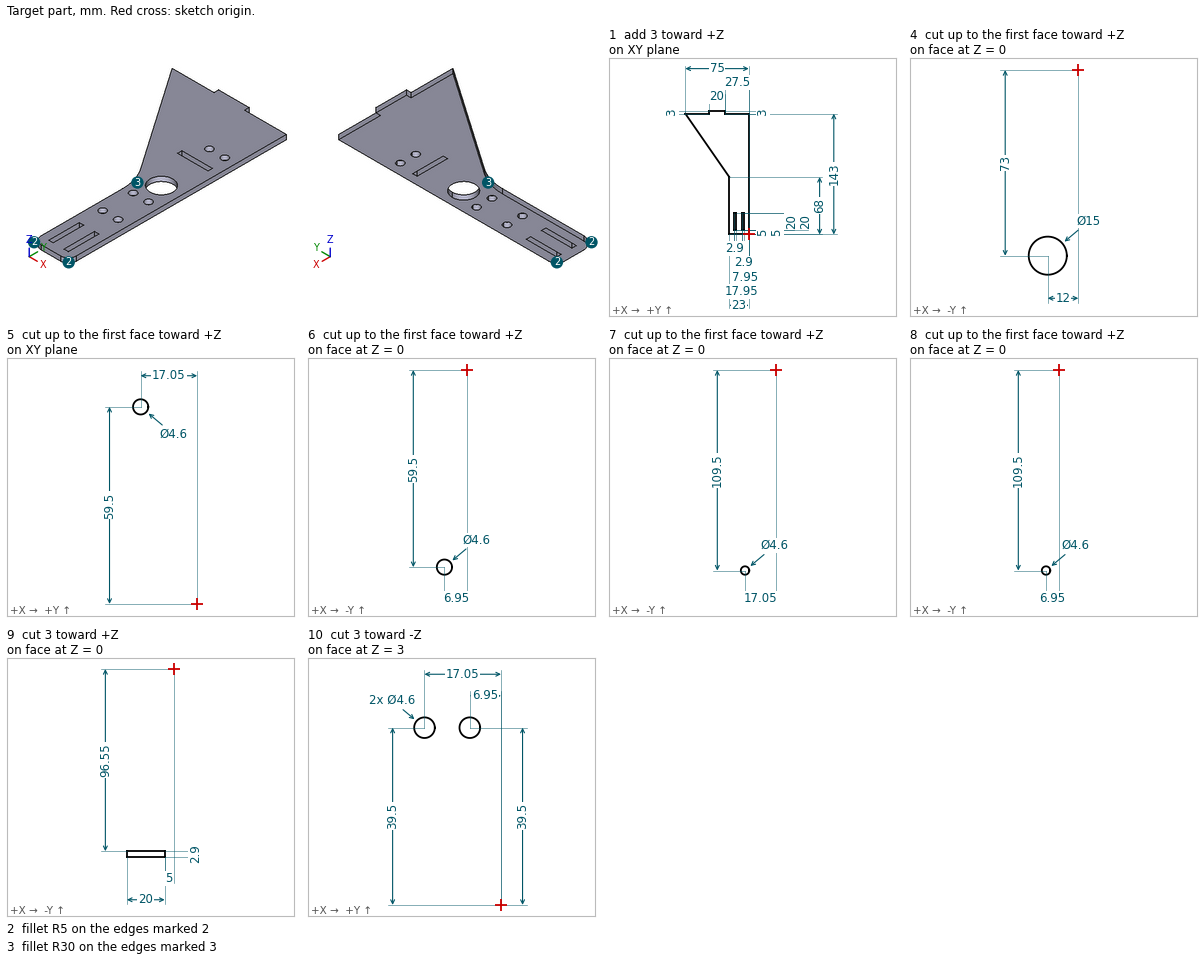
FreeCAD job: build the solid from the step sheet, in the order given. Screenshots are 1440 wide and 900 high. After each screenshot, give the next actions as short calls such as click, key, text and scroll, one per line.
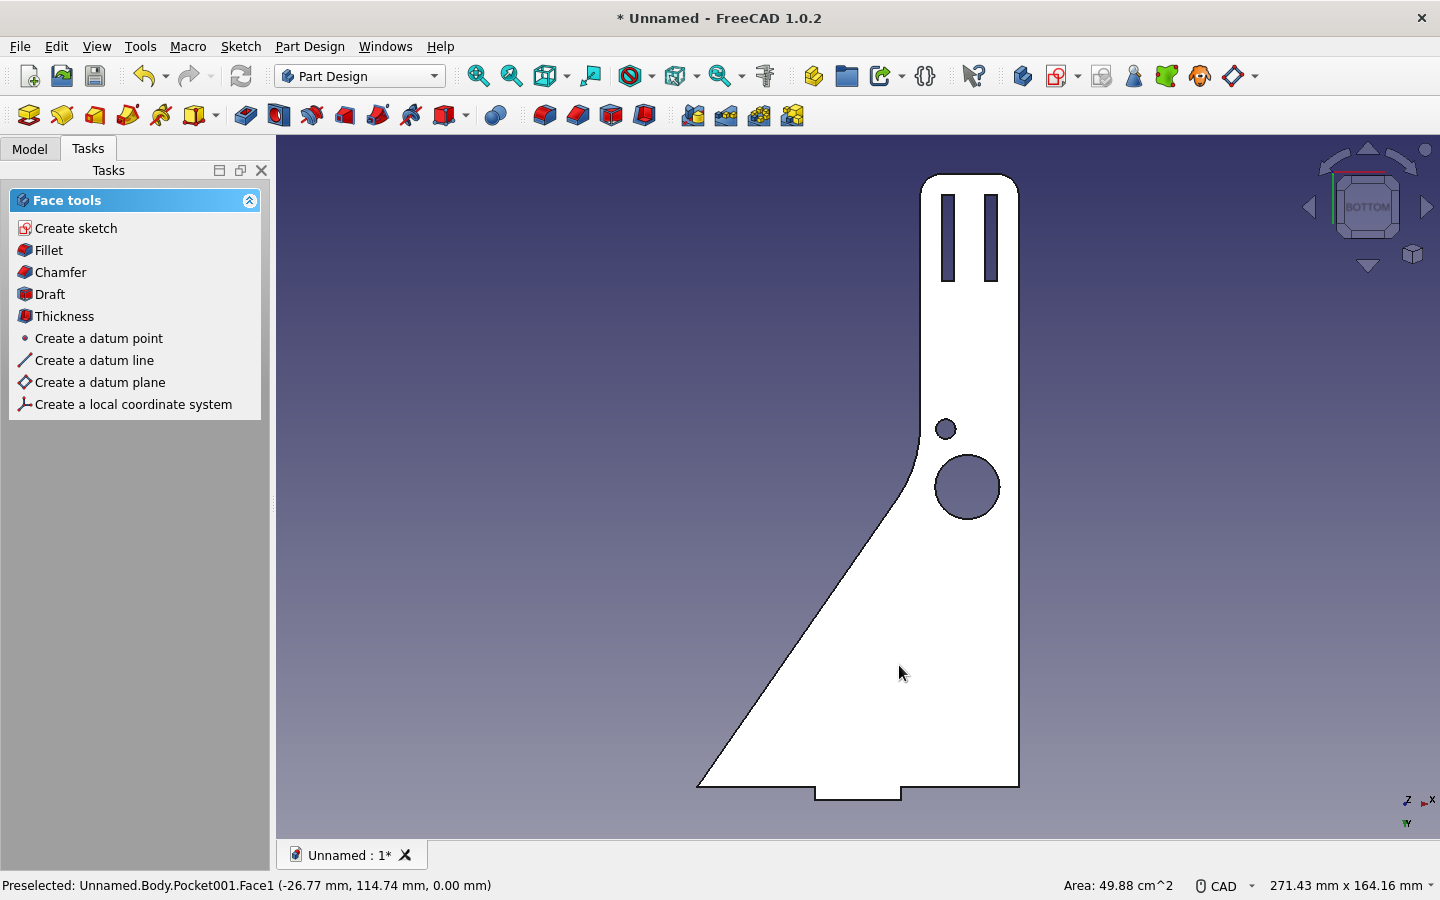
click(1056, 76)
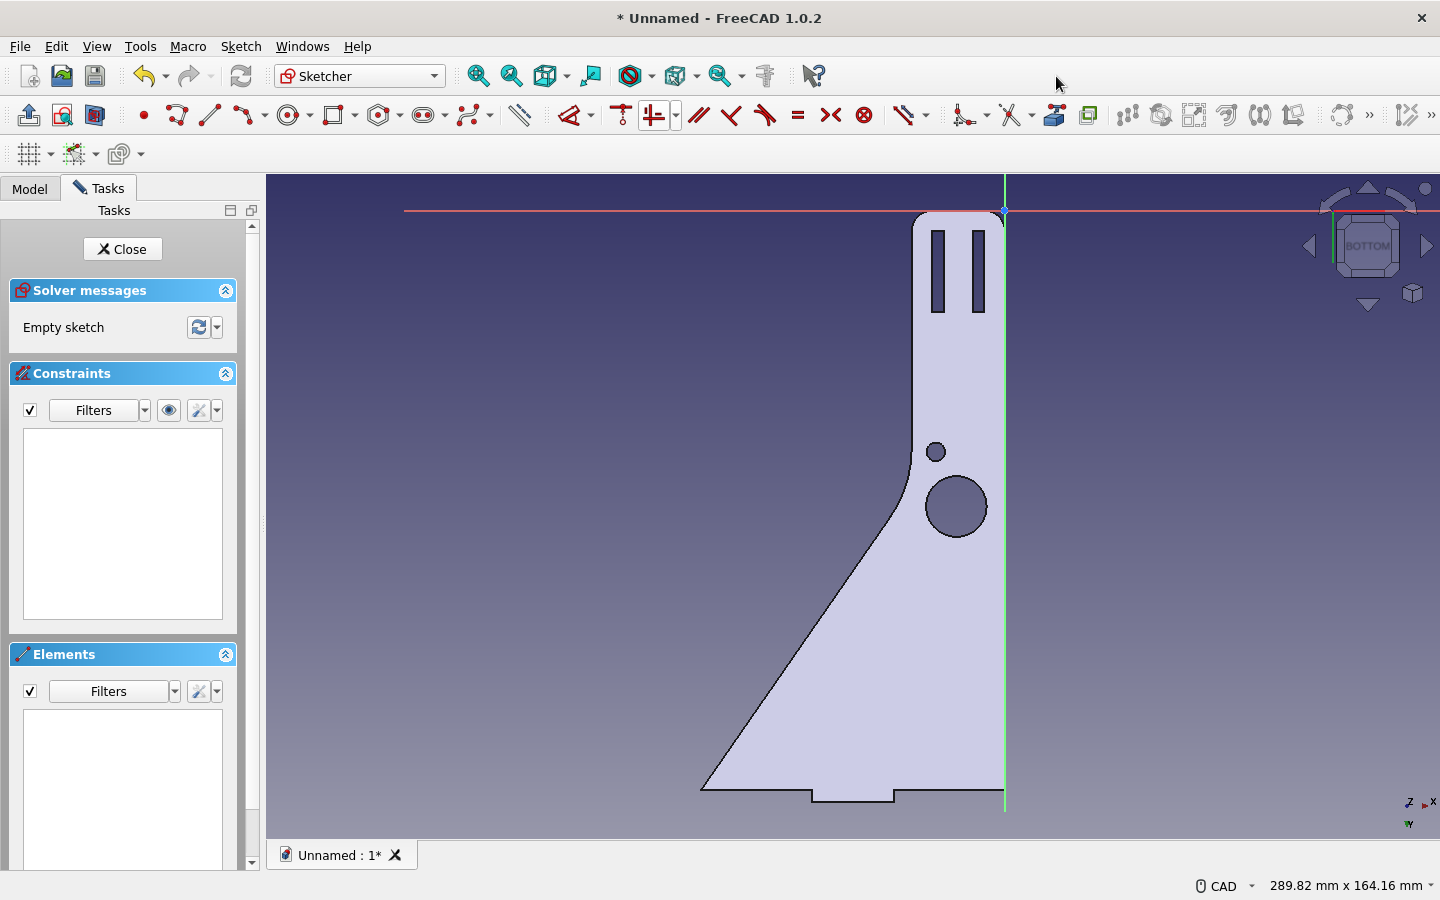
scroll(987, 449, up, 15)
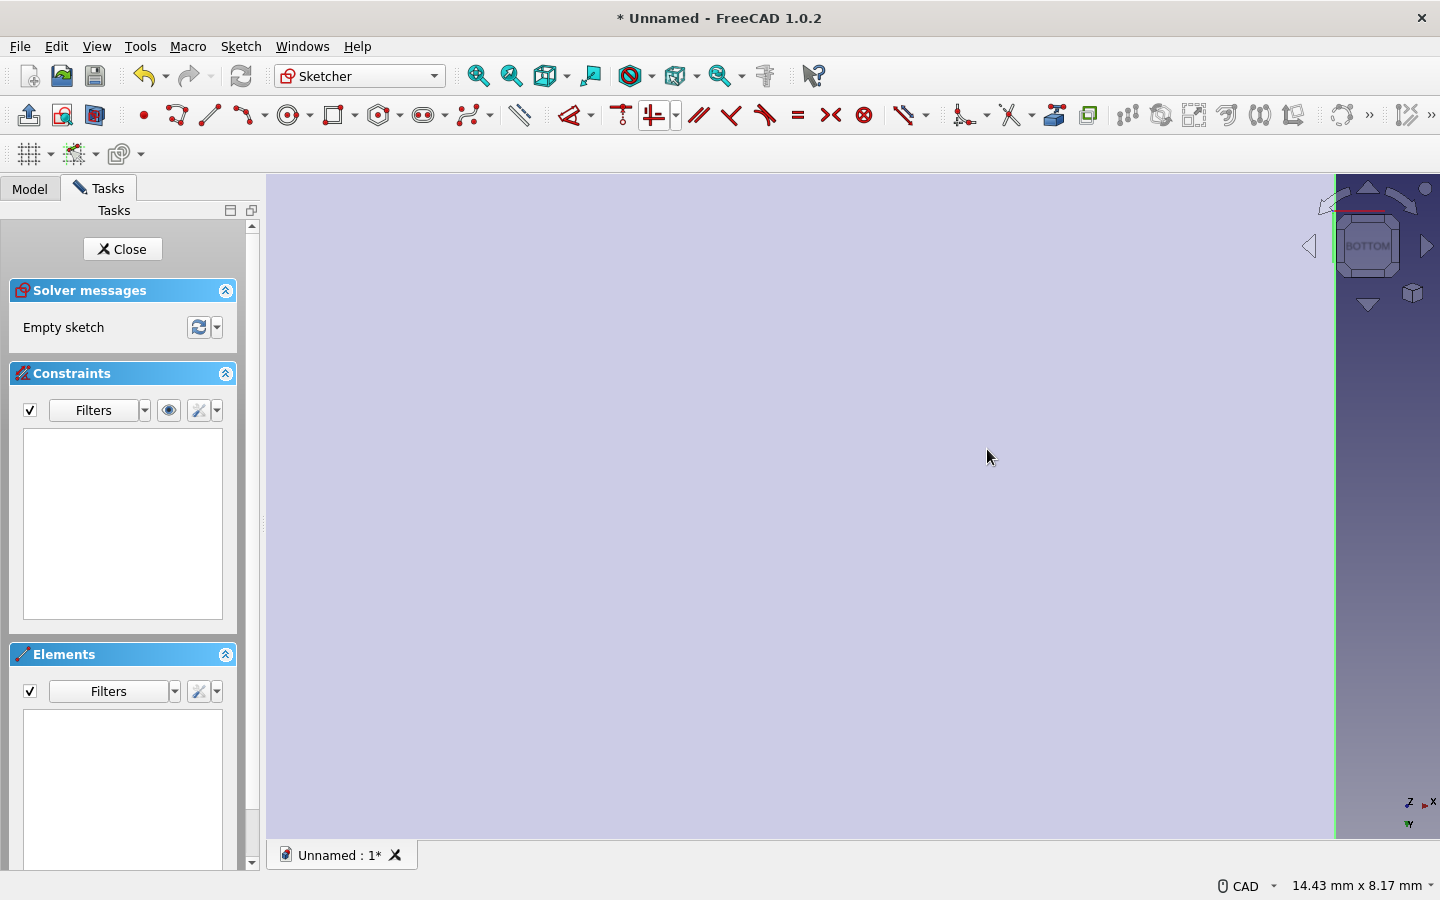
key(g)
key(c)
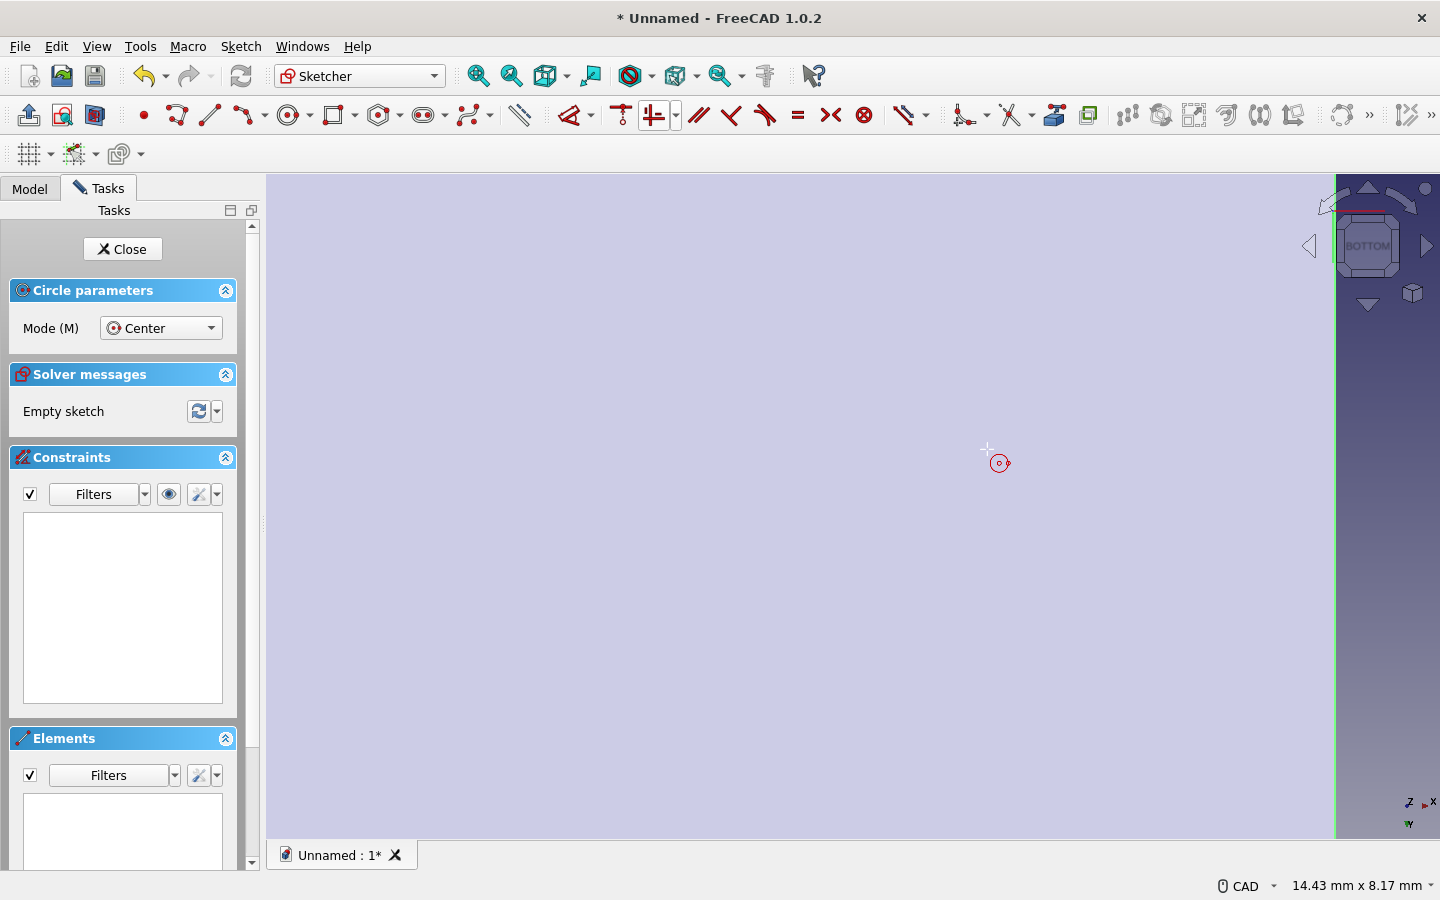
click(769, 498)
move(902, 365)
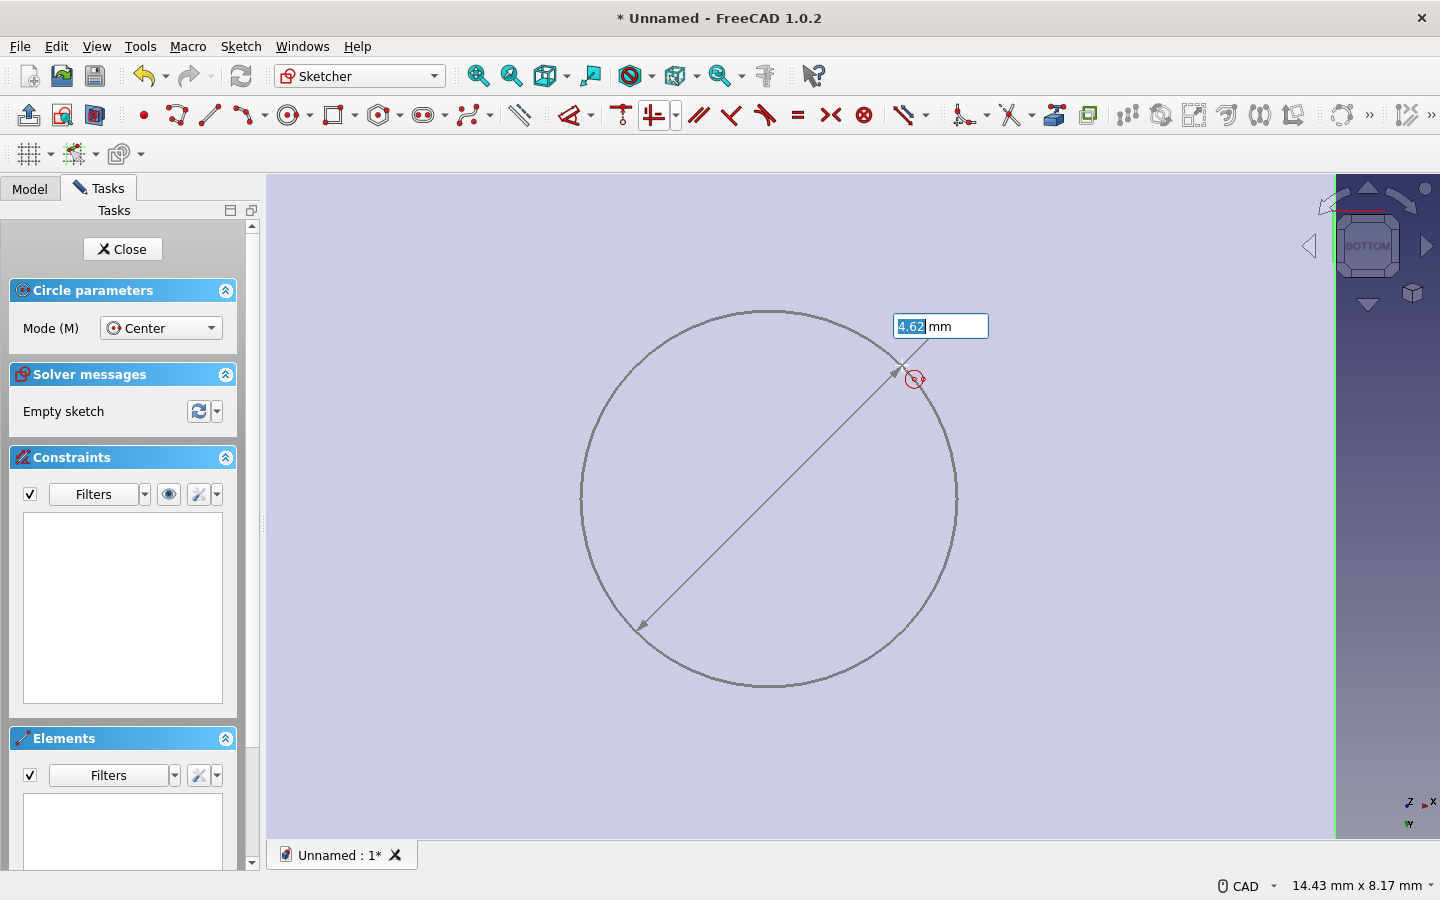
text(4.6)
key(Return)
key(Escape)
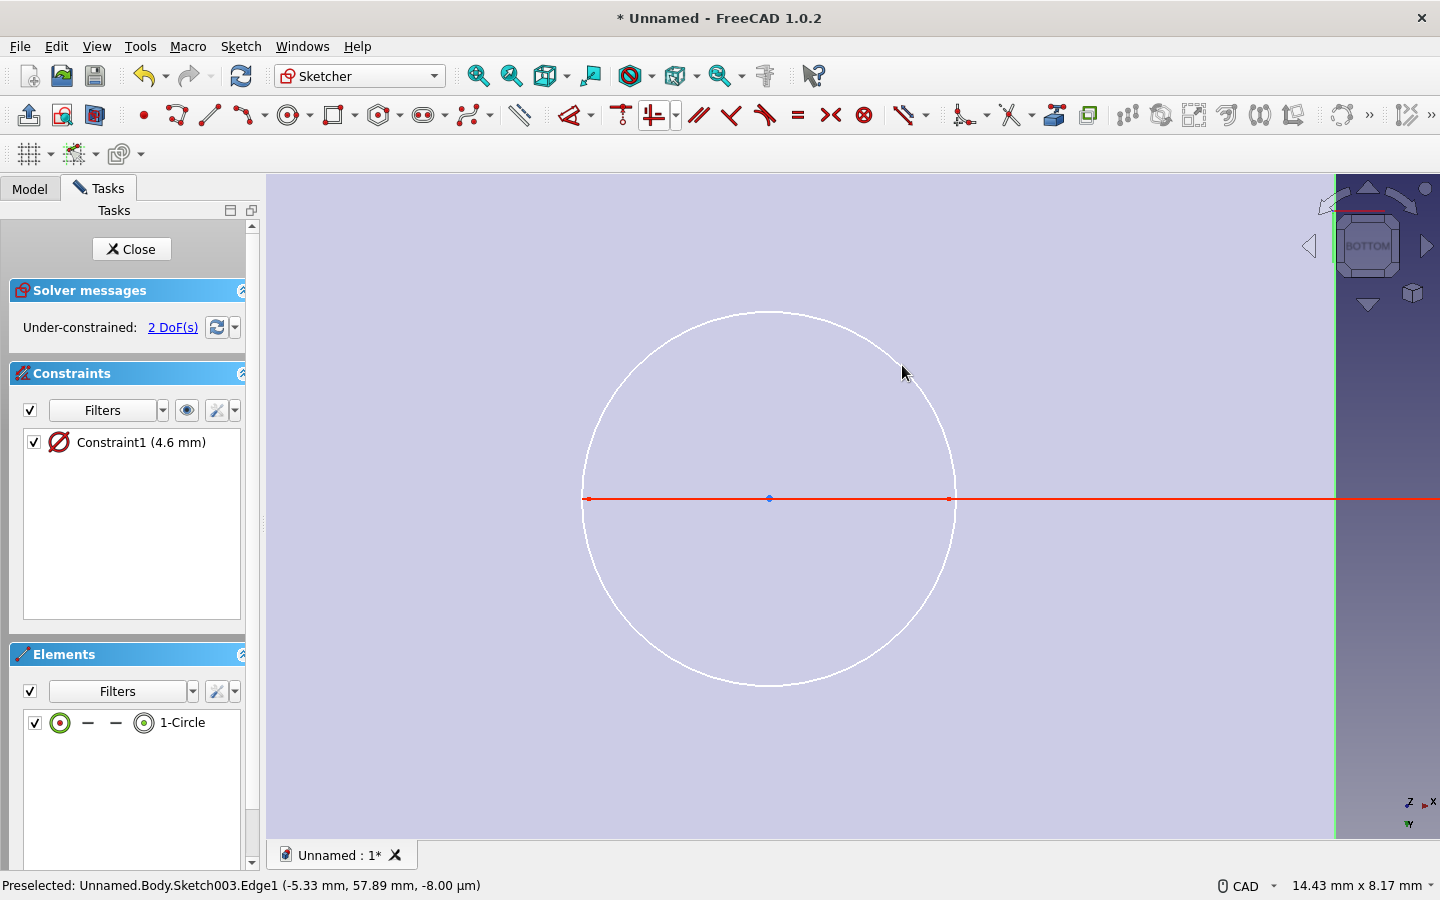
click(568, 116)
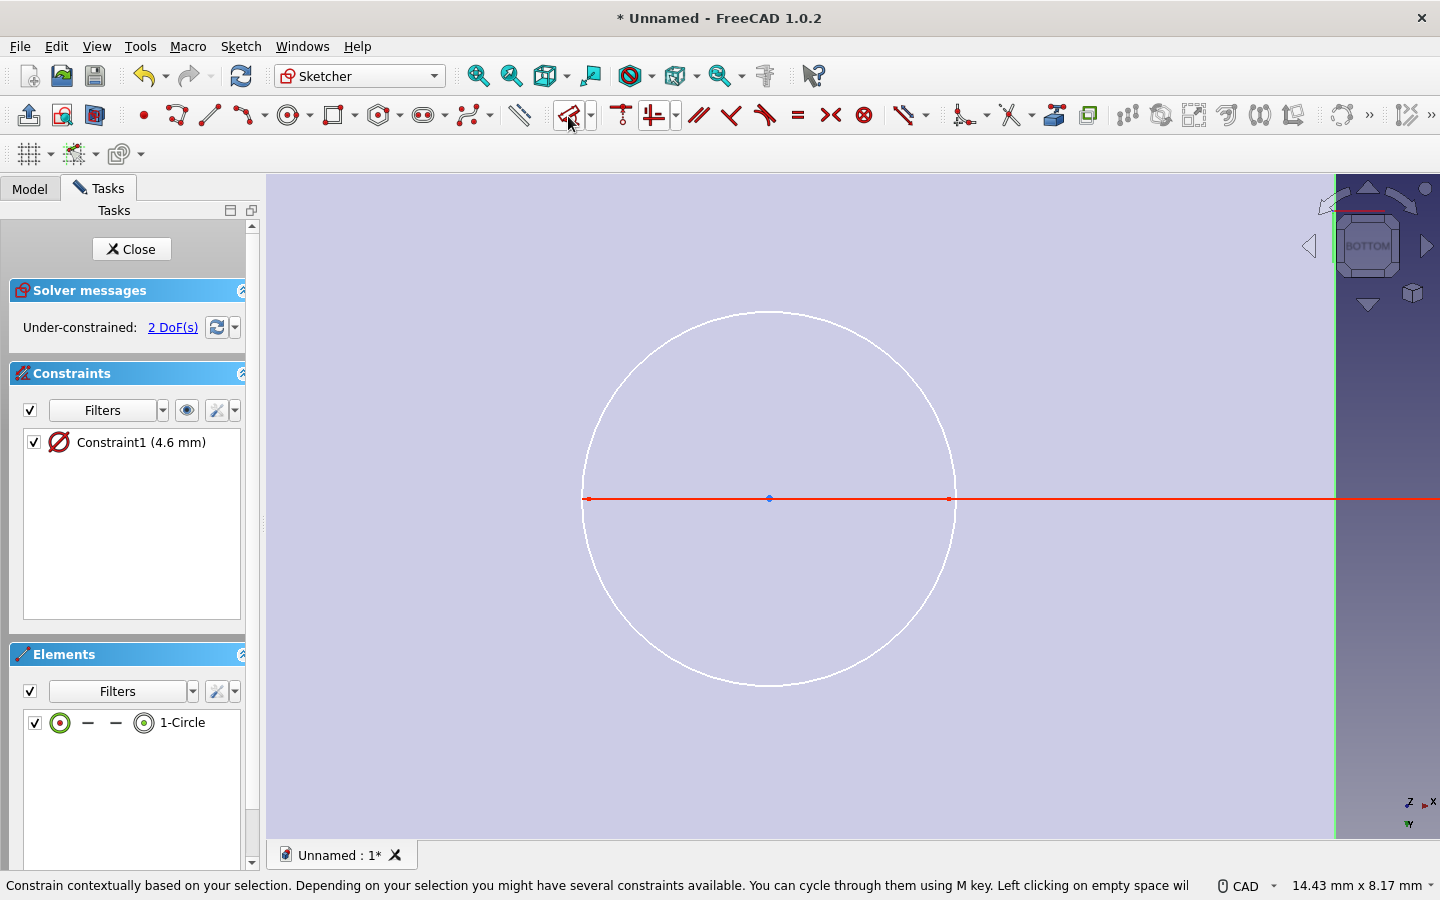
click(769, 499)
click(1022, 533)